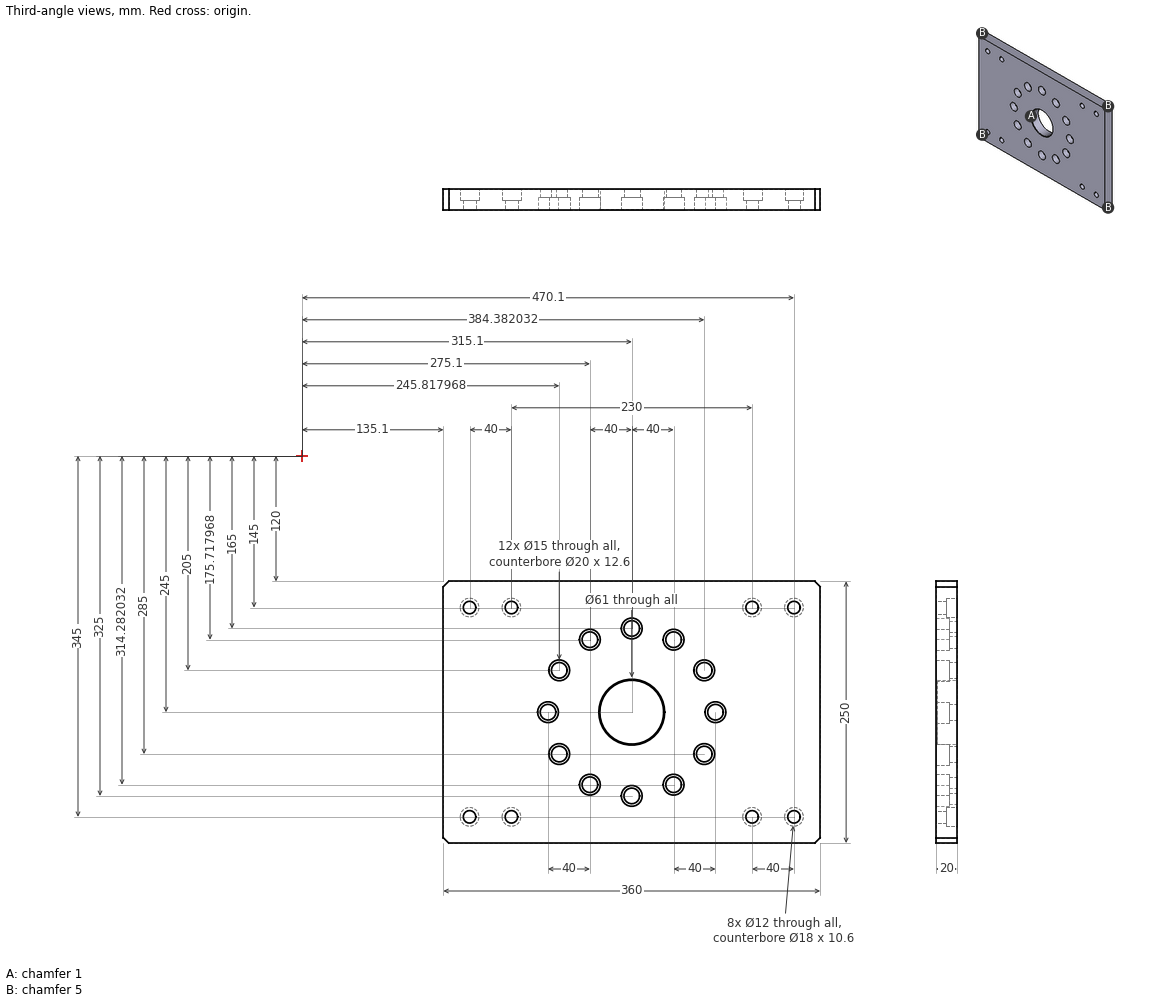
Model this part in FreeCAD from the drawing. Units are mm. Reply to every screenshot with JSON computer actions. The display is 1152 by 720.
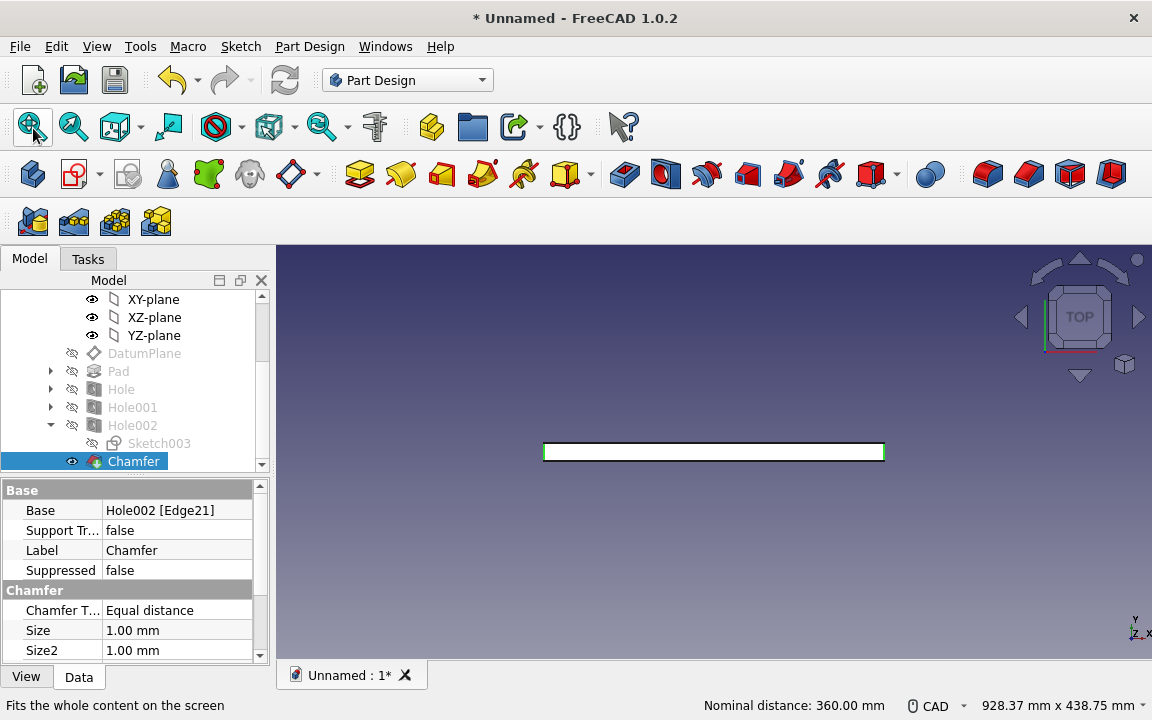
{"action": "key", "text": "0"}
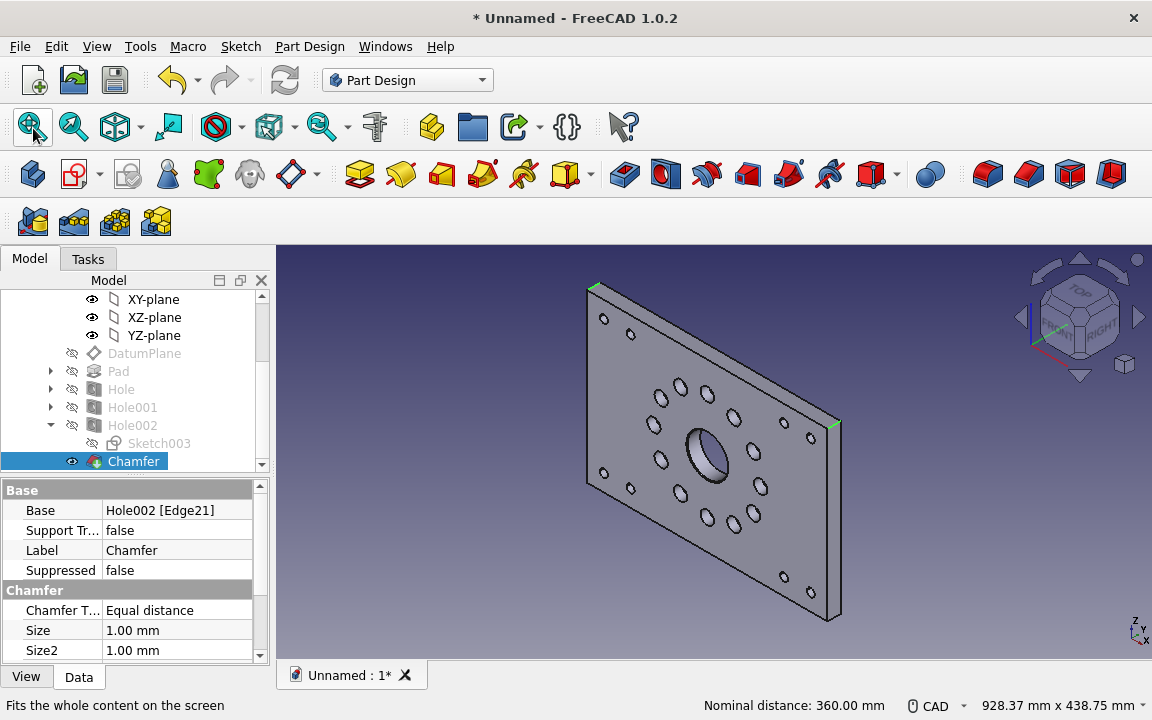
{"action": "scroll", "coordinate": [834, 617], "scroll_direction": "up", "scroll_amount": 4}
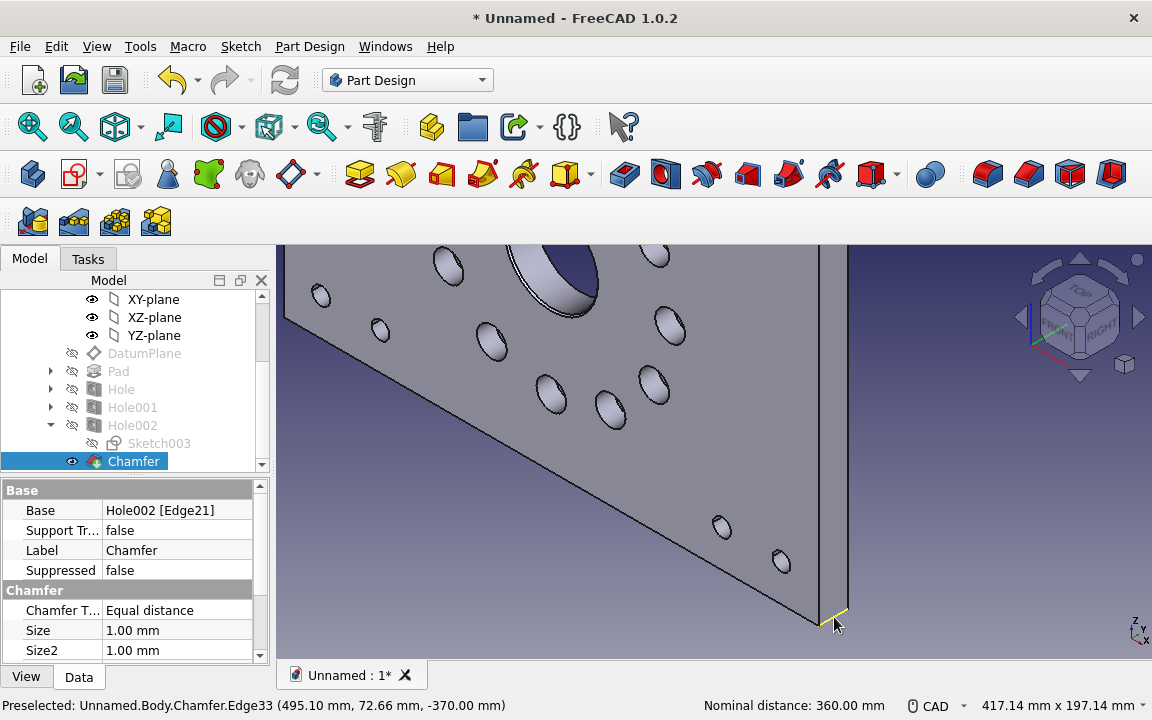
{"action": "left_click", "coordinate": [33, 128]}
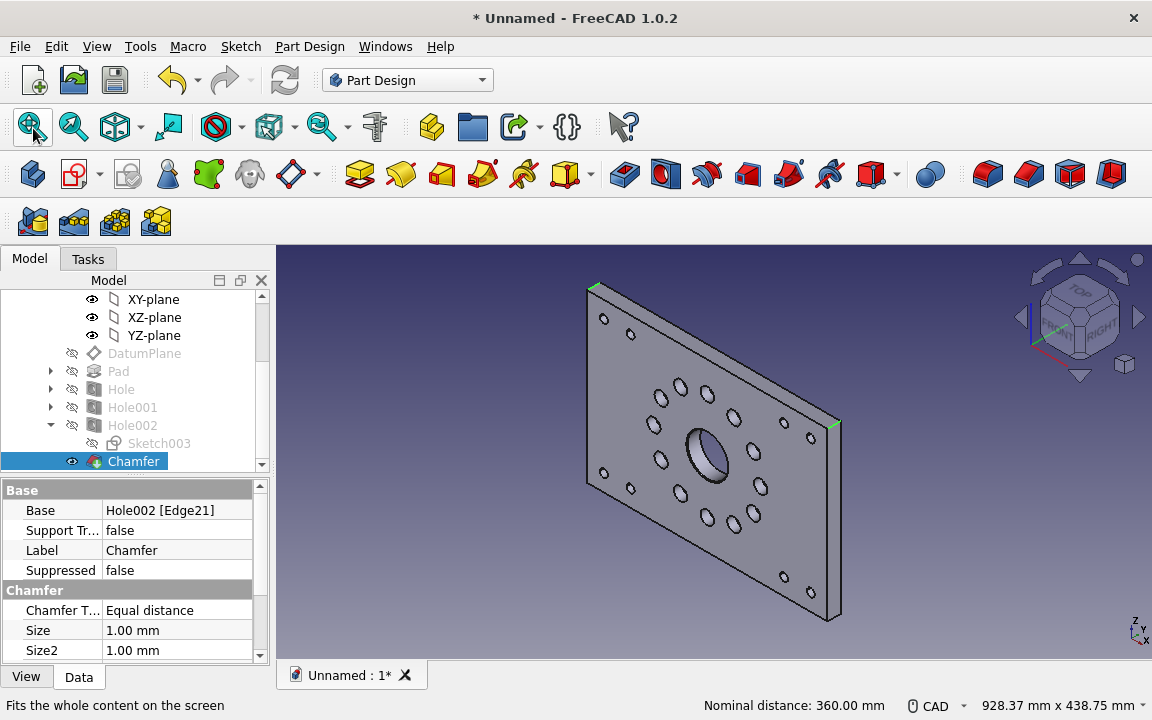
{"action": "key", "text": "1"}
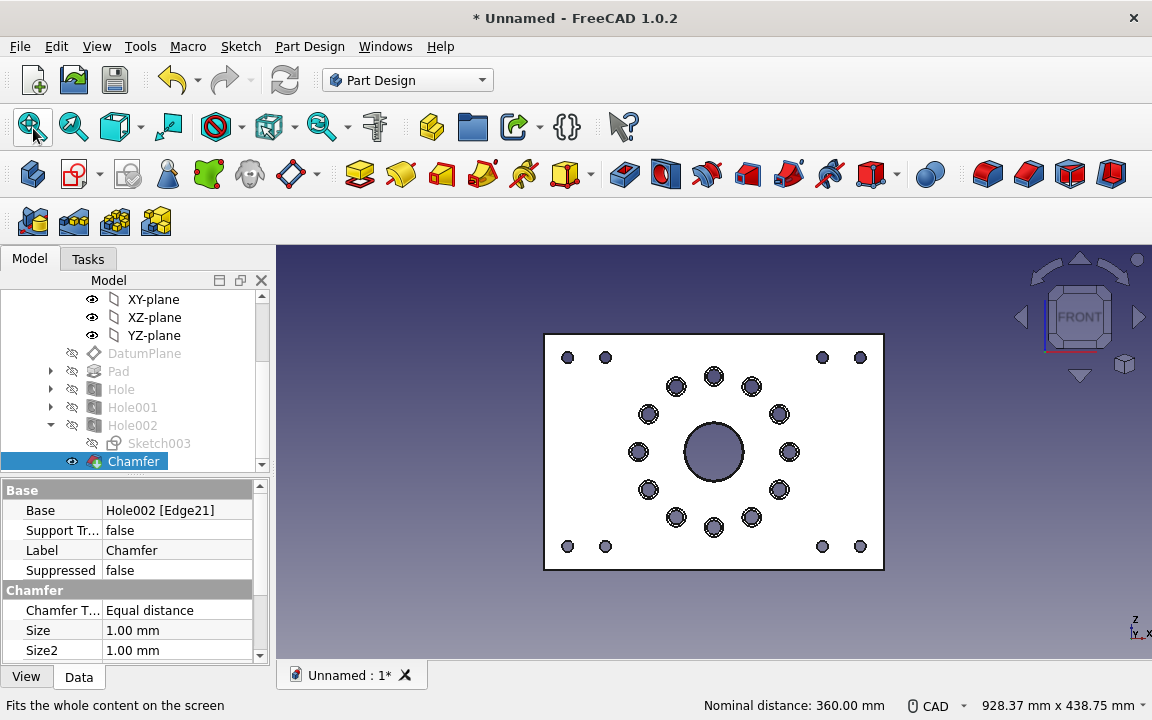
{"action": "scroll", "coordinate": [884, 569], "scroll_direction": "up", "scroll_amount": 4}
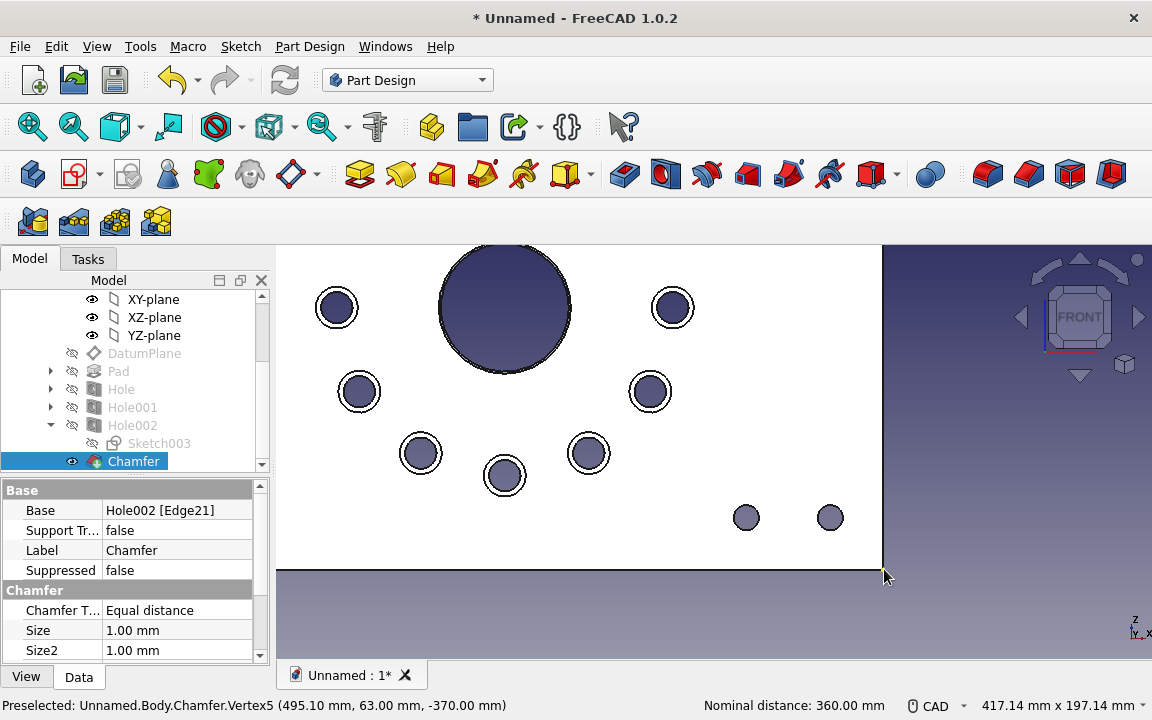
{"action": "left_click", "coordinate": [33, 128]}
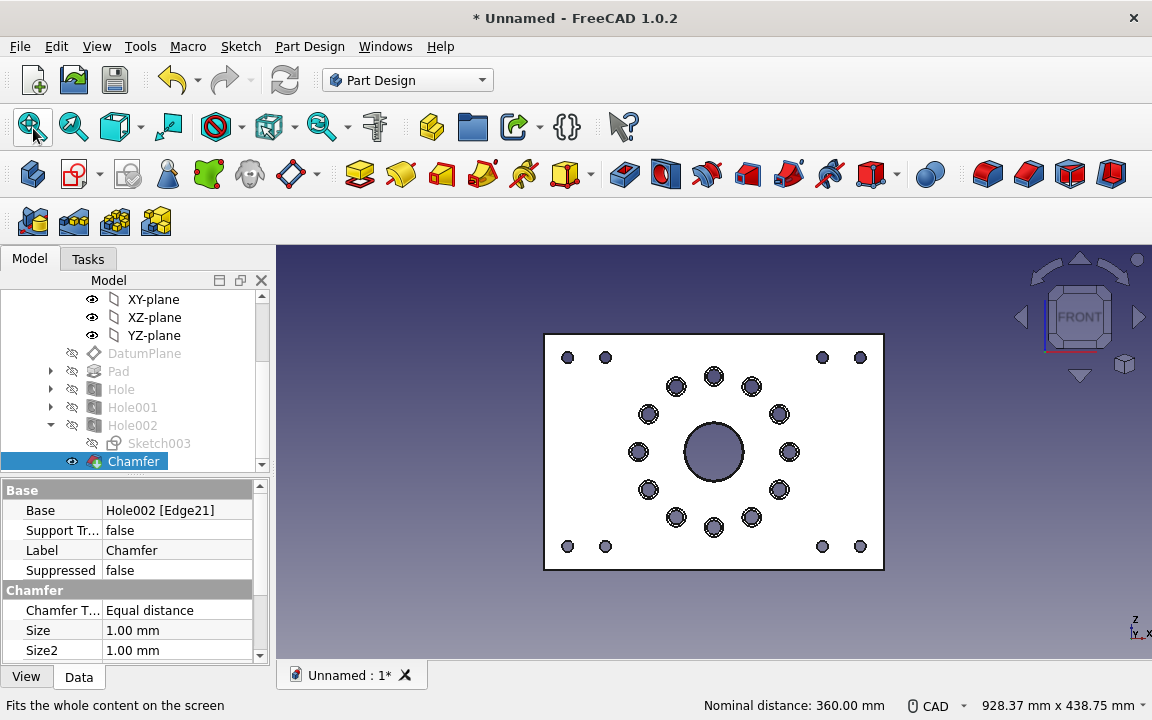
{"action": "key", "text": "3"}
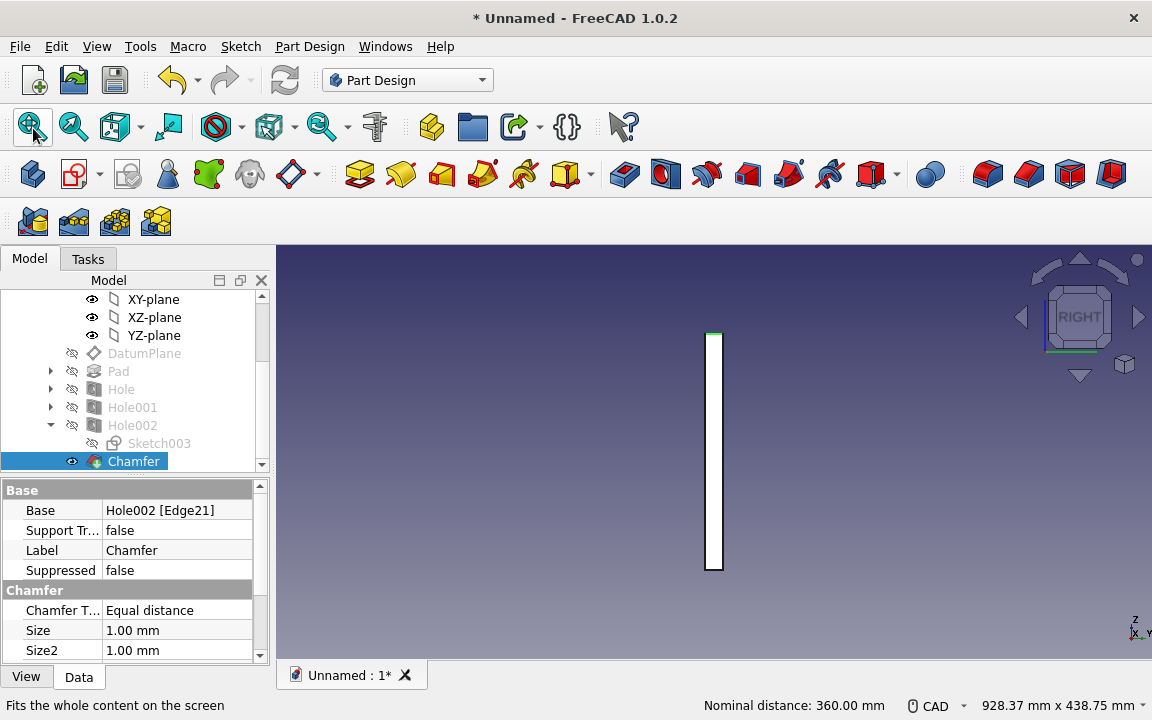
{"action": "left_click", "coordinate": [714, 569], "text": "ctrl"}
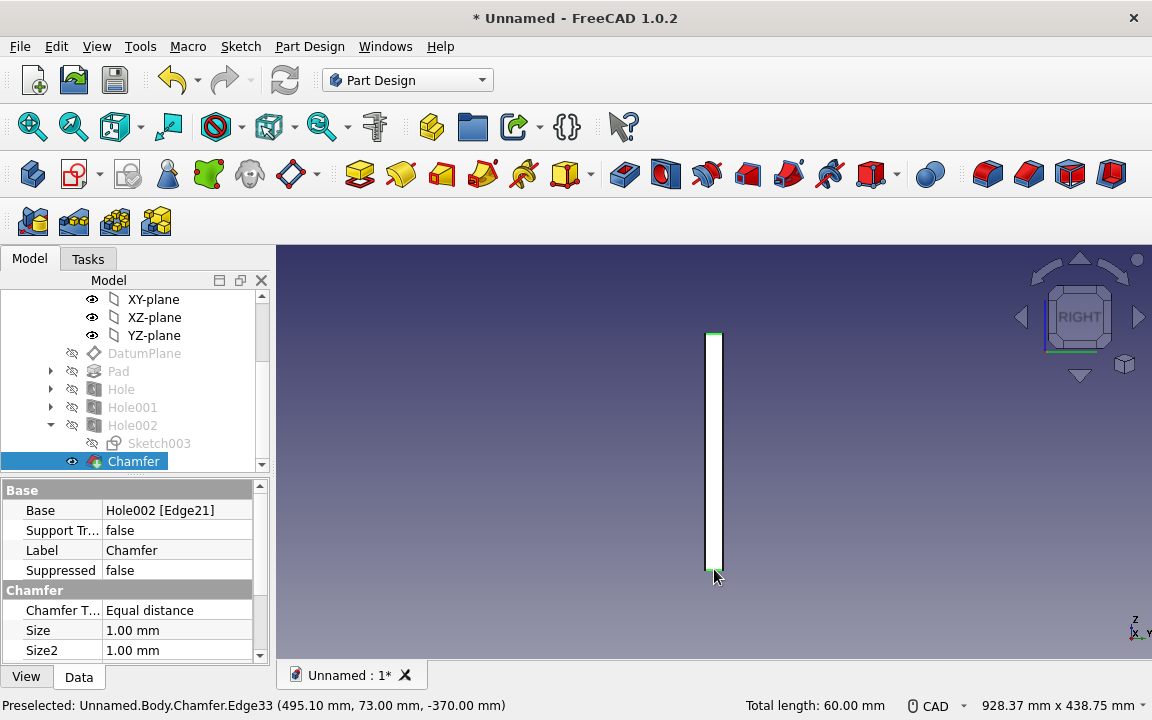
{"action": "scroll", "coordinate": [714, 569], "scroll_direction": "up", "scroll_amount": 4}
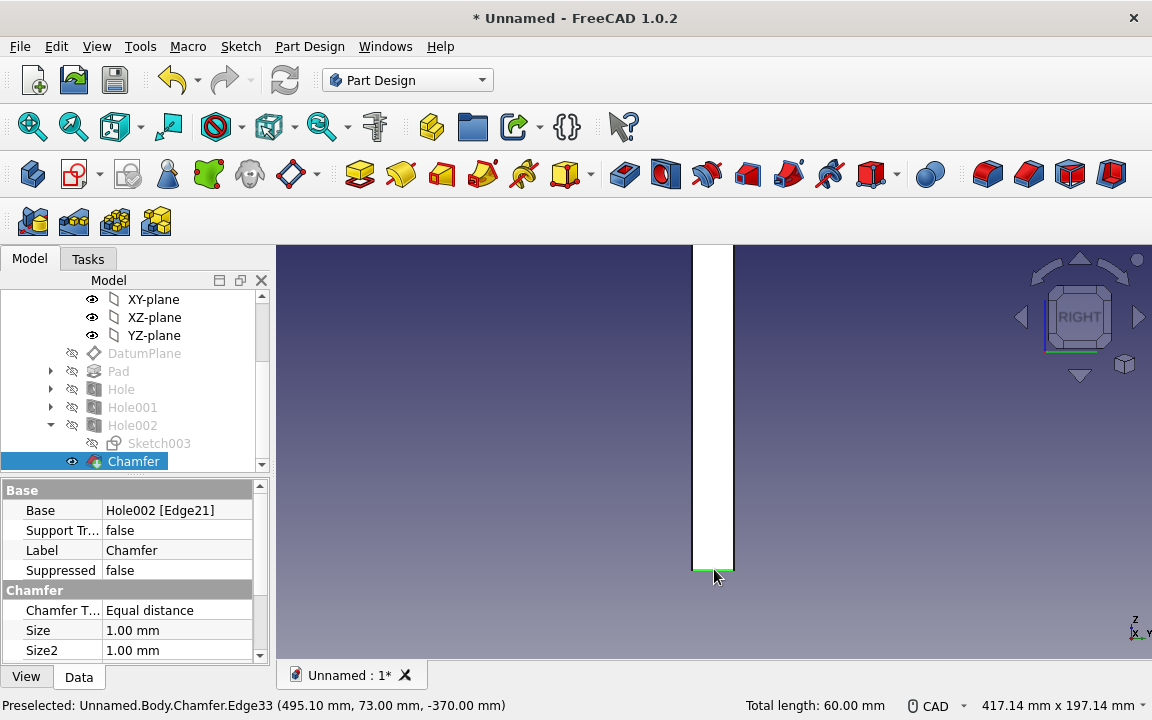
{"action": "left_click", "coordinate": [33, 128]}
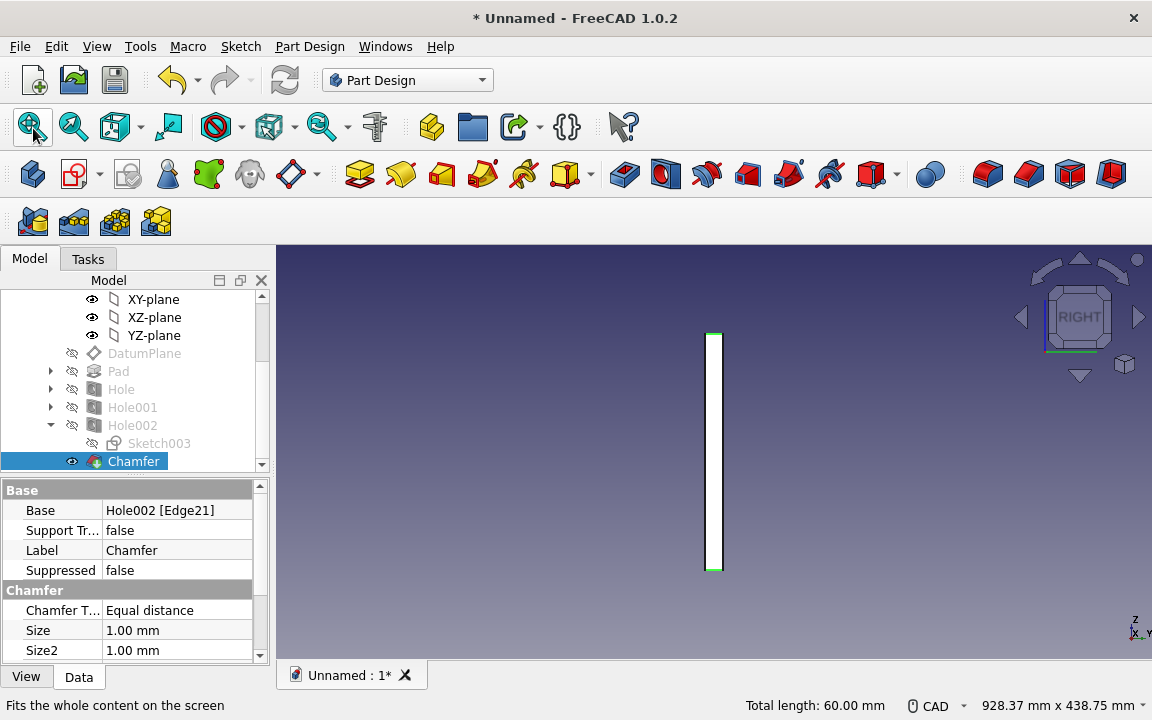
{"action": "key", "text": "5"}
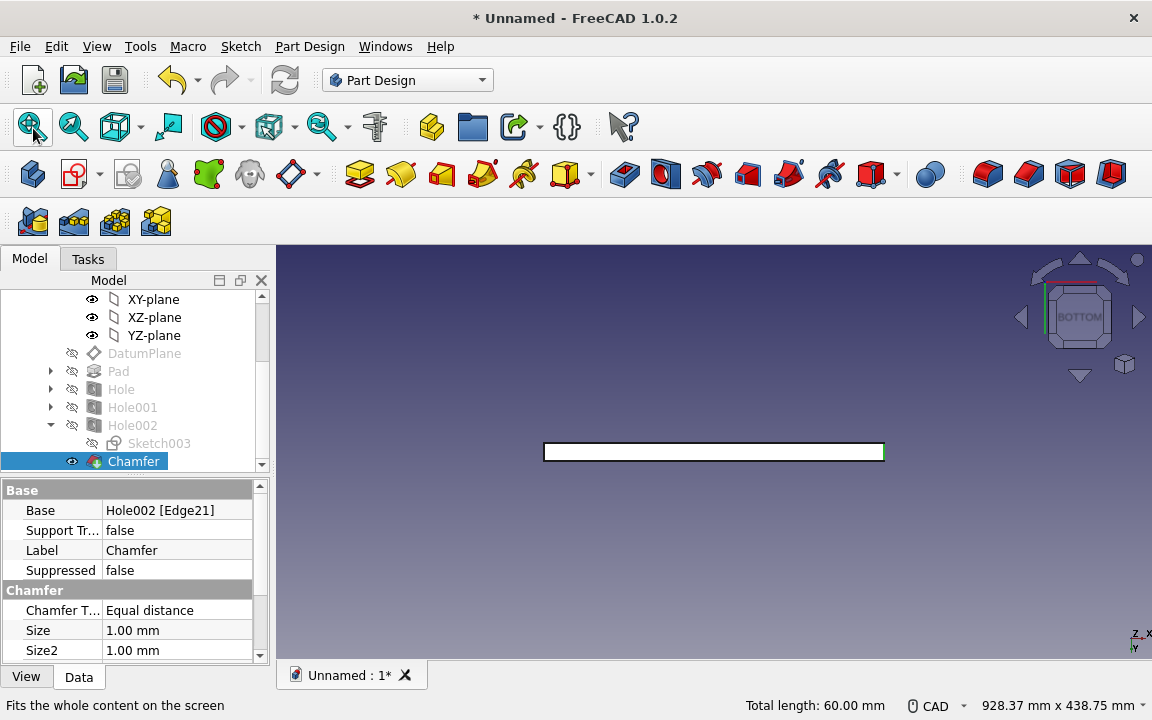
{"action": "left_click", "coordinate": [33, 128]}